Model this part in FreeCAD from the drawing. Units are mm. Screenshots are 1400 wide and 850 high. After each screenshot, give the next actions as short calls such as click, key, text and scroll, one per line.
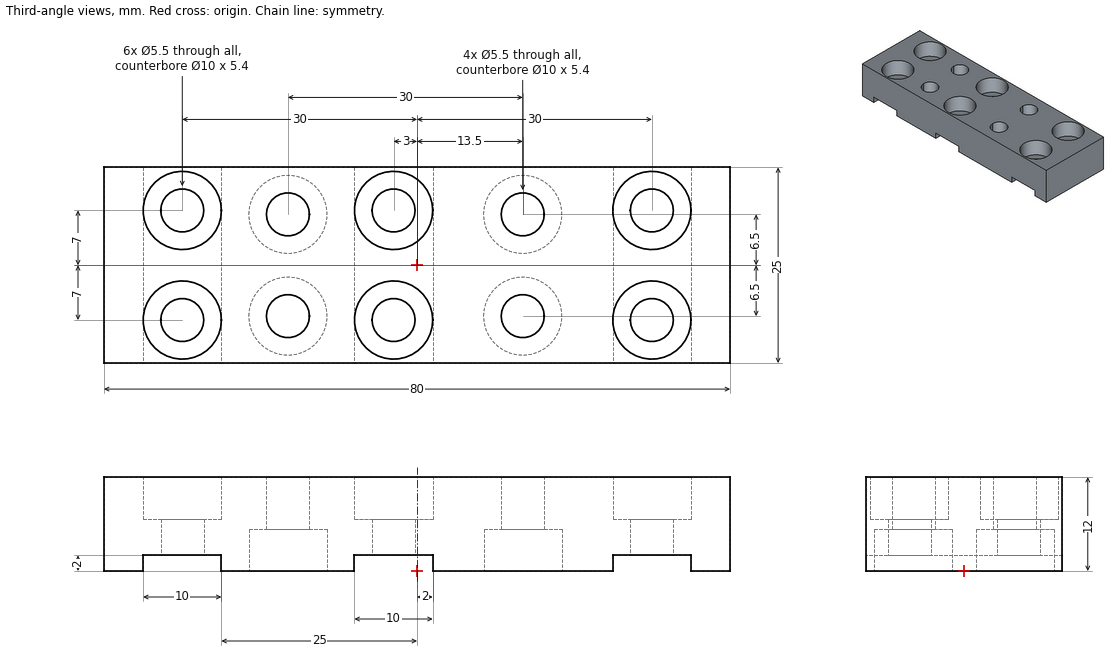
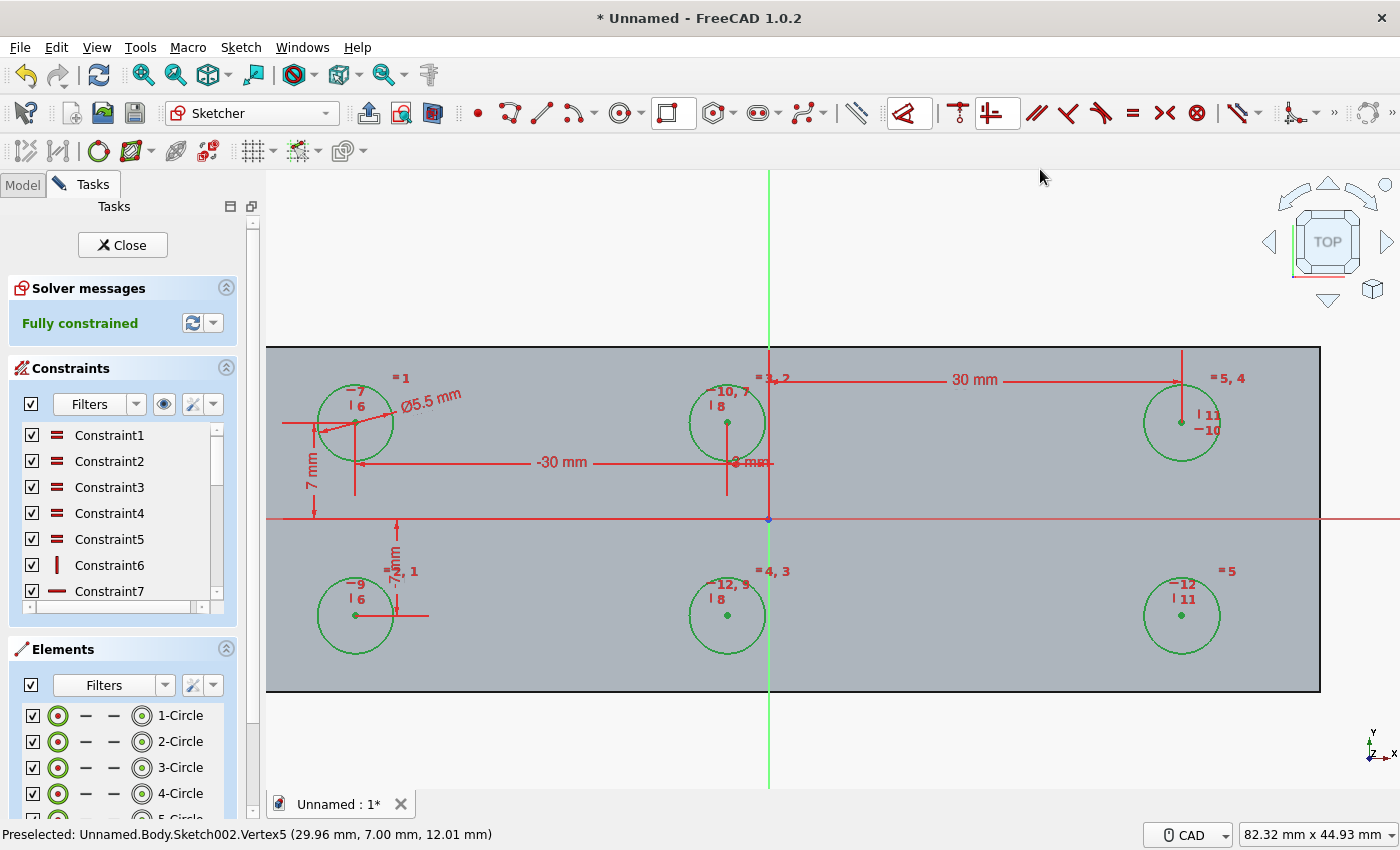
click(123, 245)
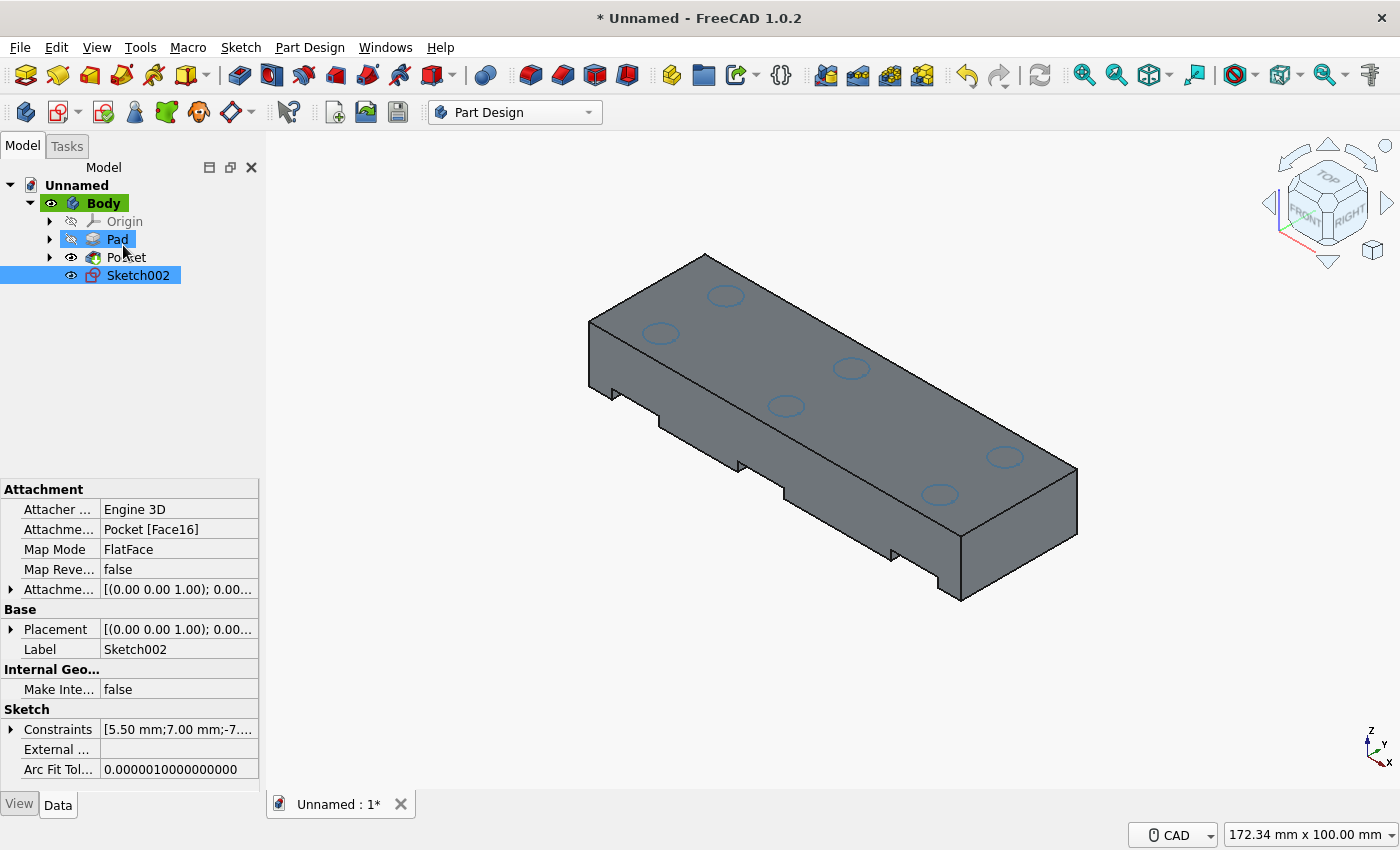
click(272, 76)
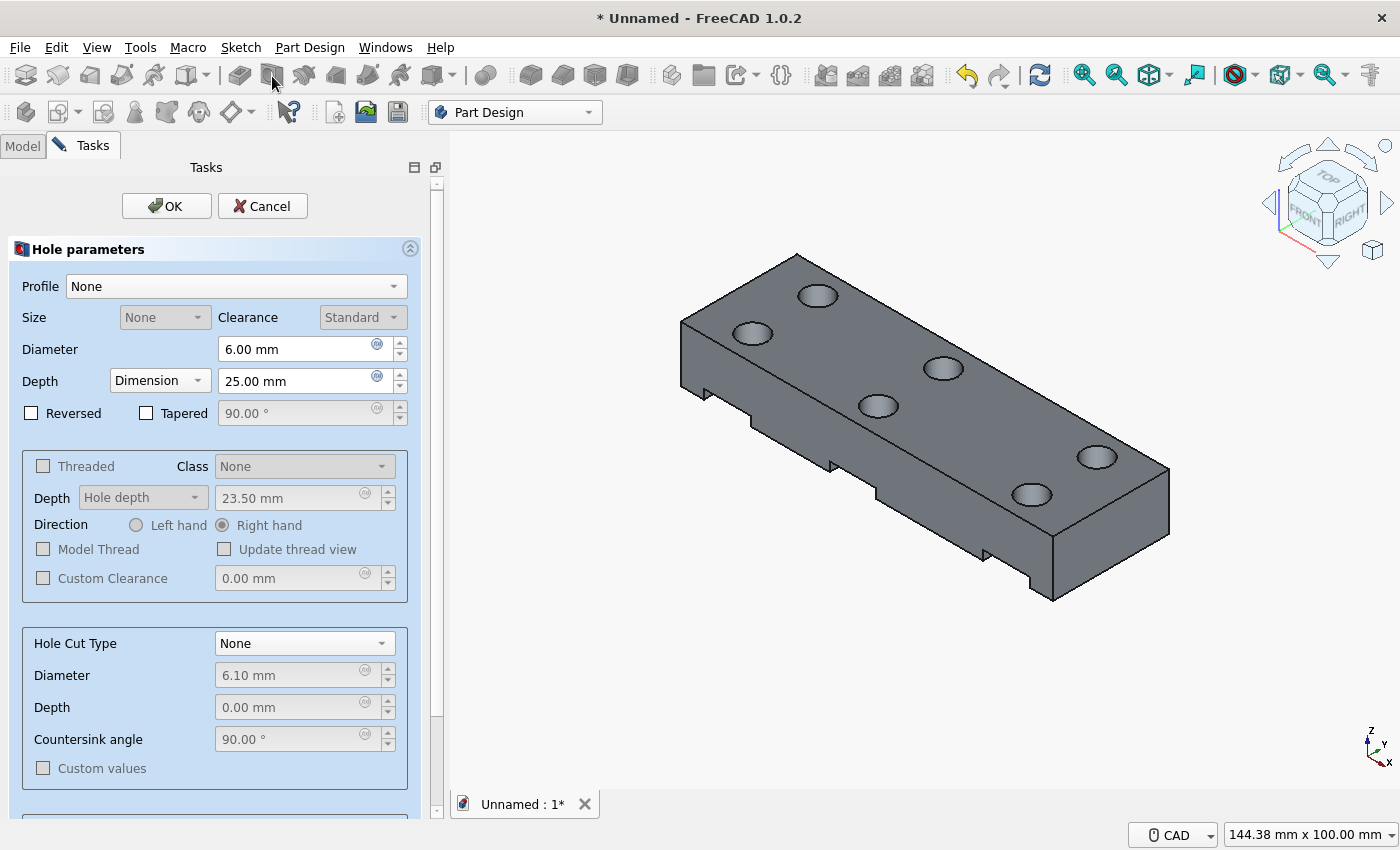
triple_click(305, 349)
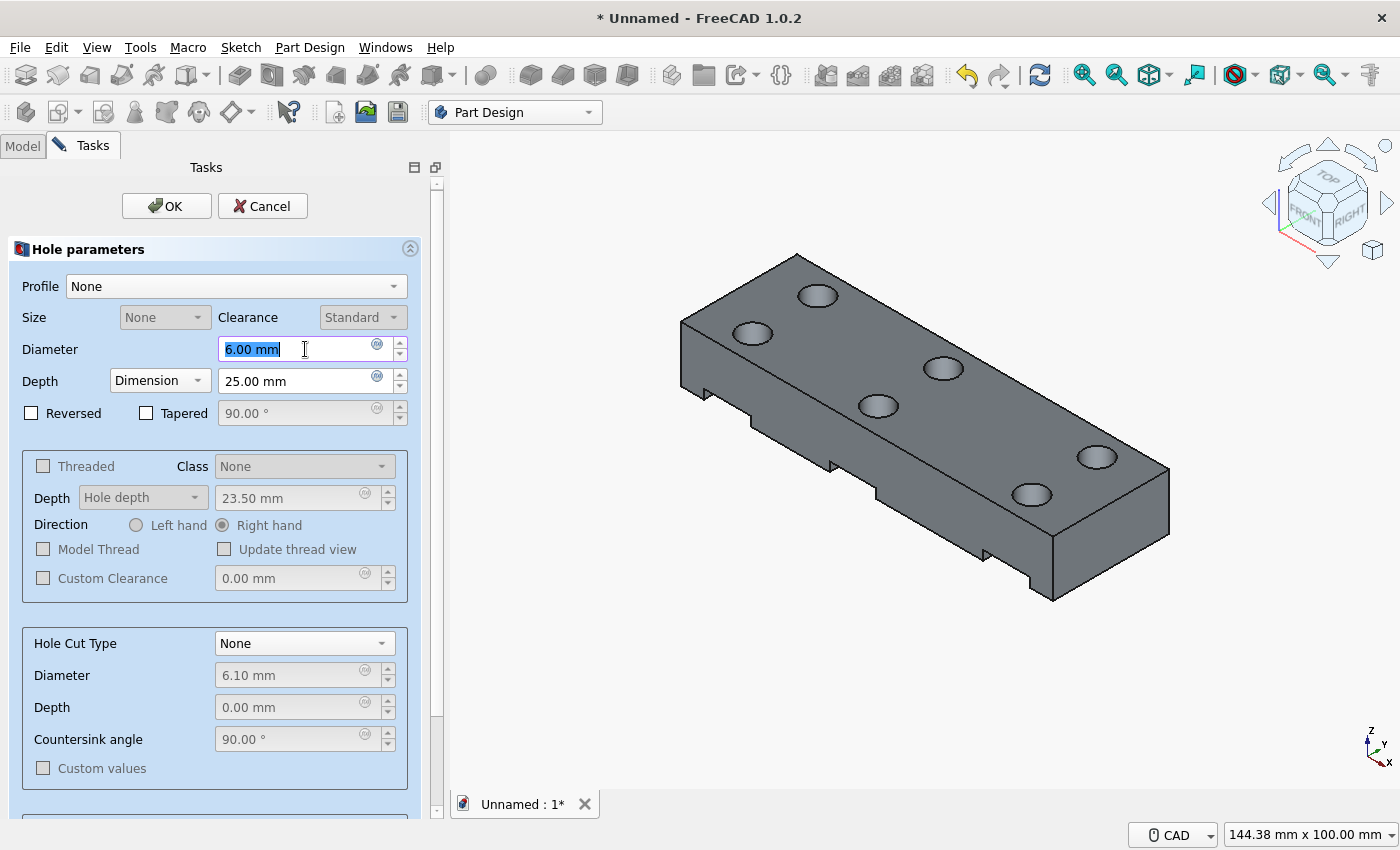
text(5.5)
key(Tab)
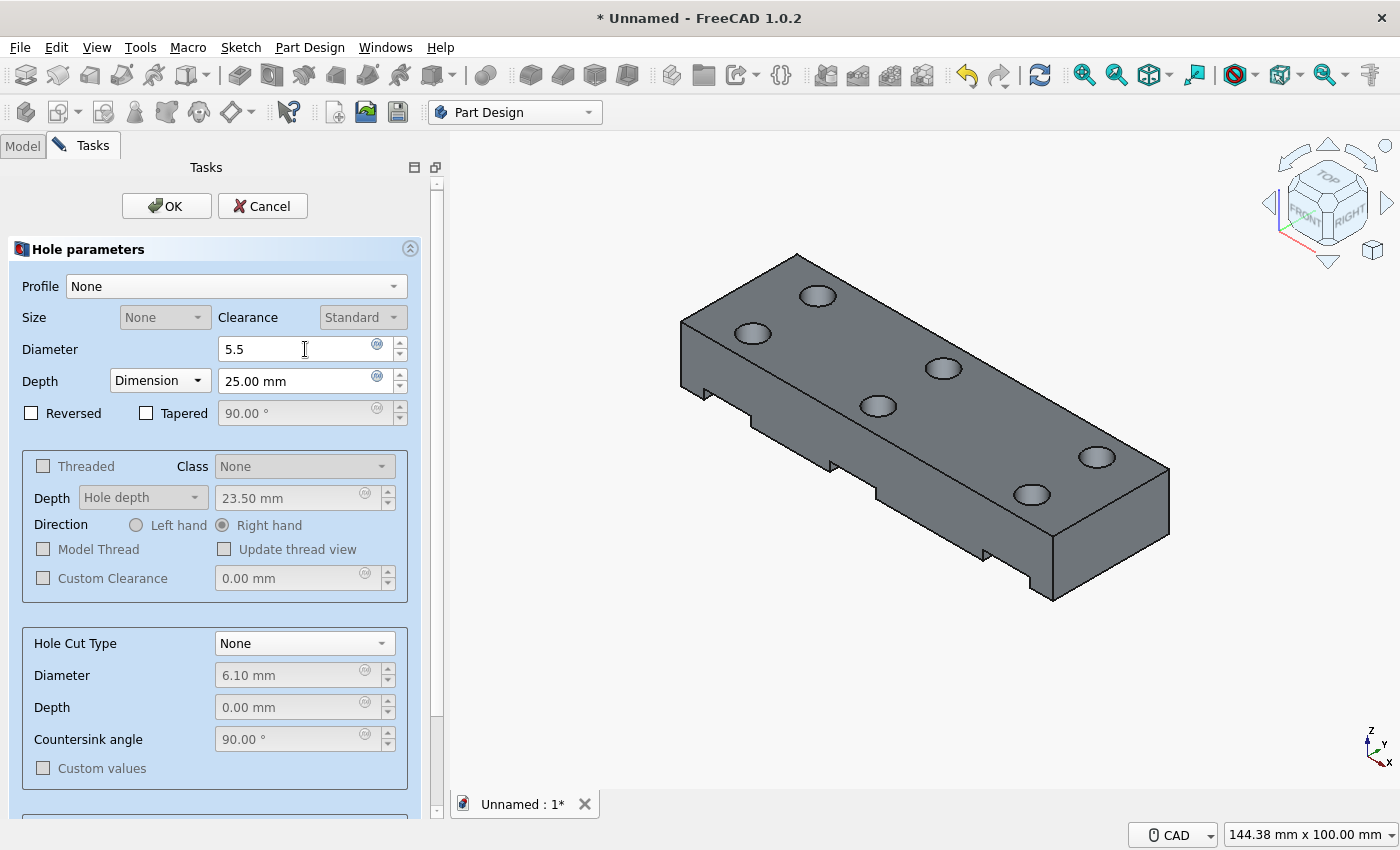
click(161, 380)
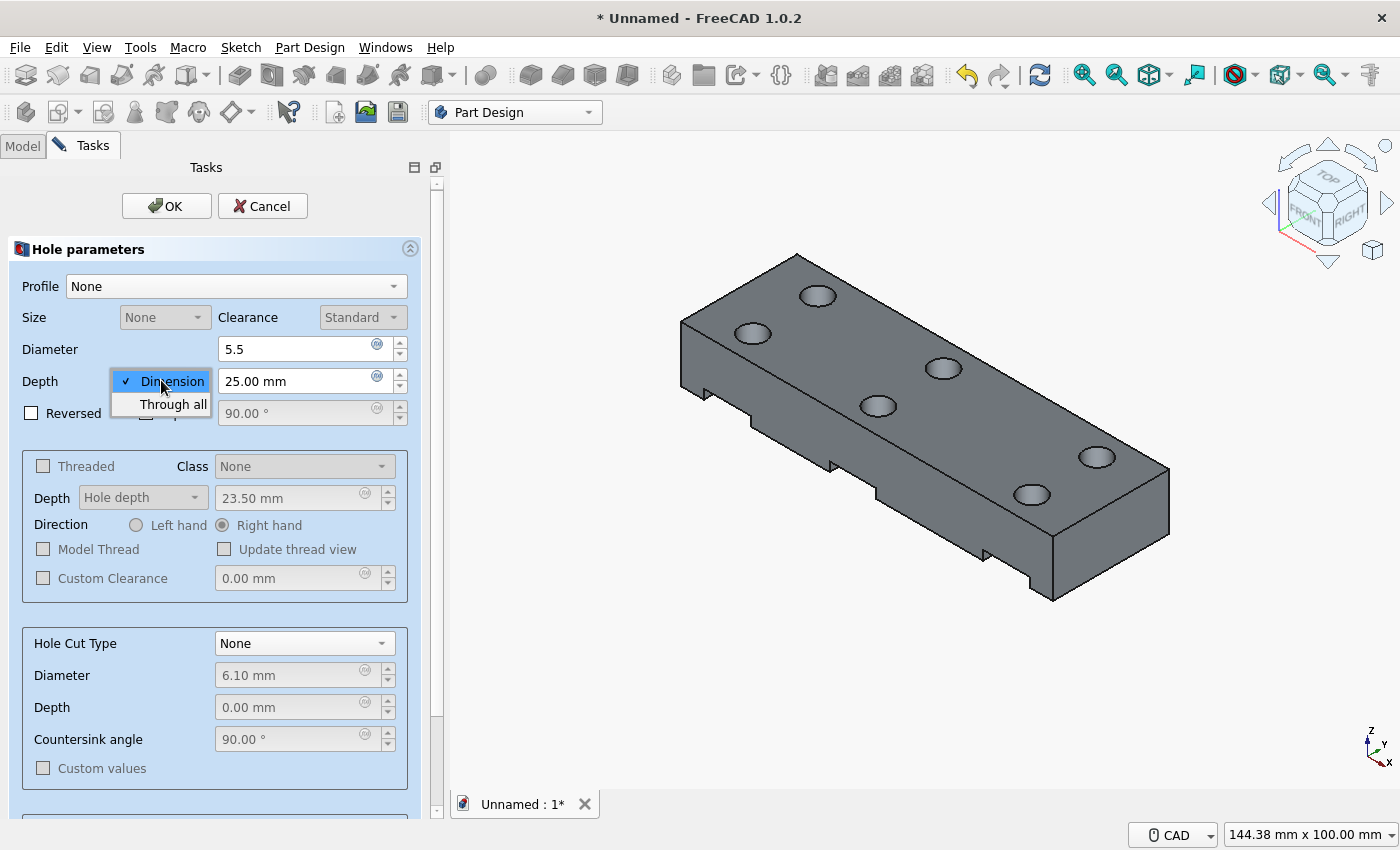
click(160, 404)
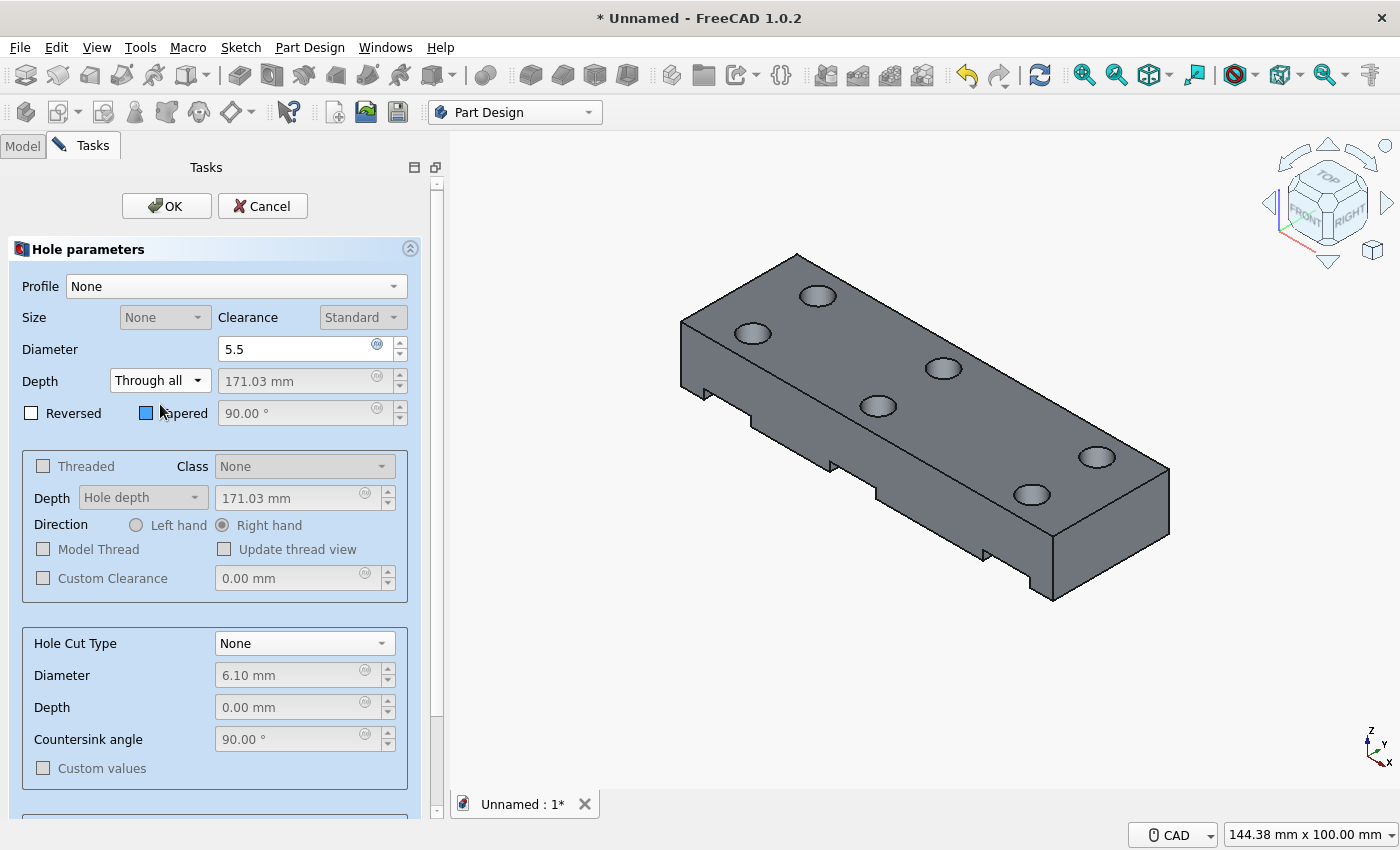
click(306, 644)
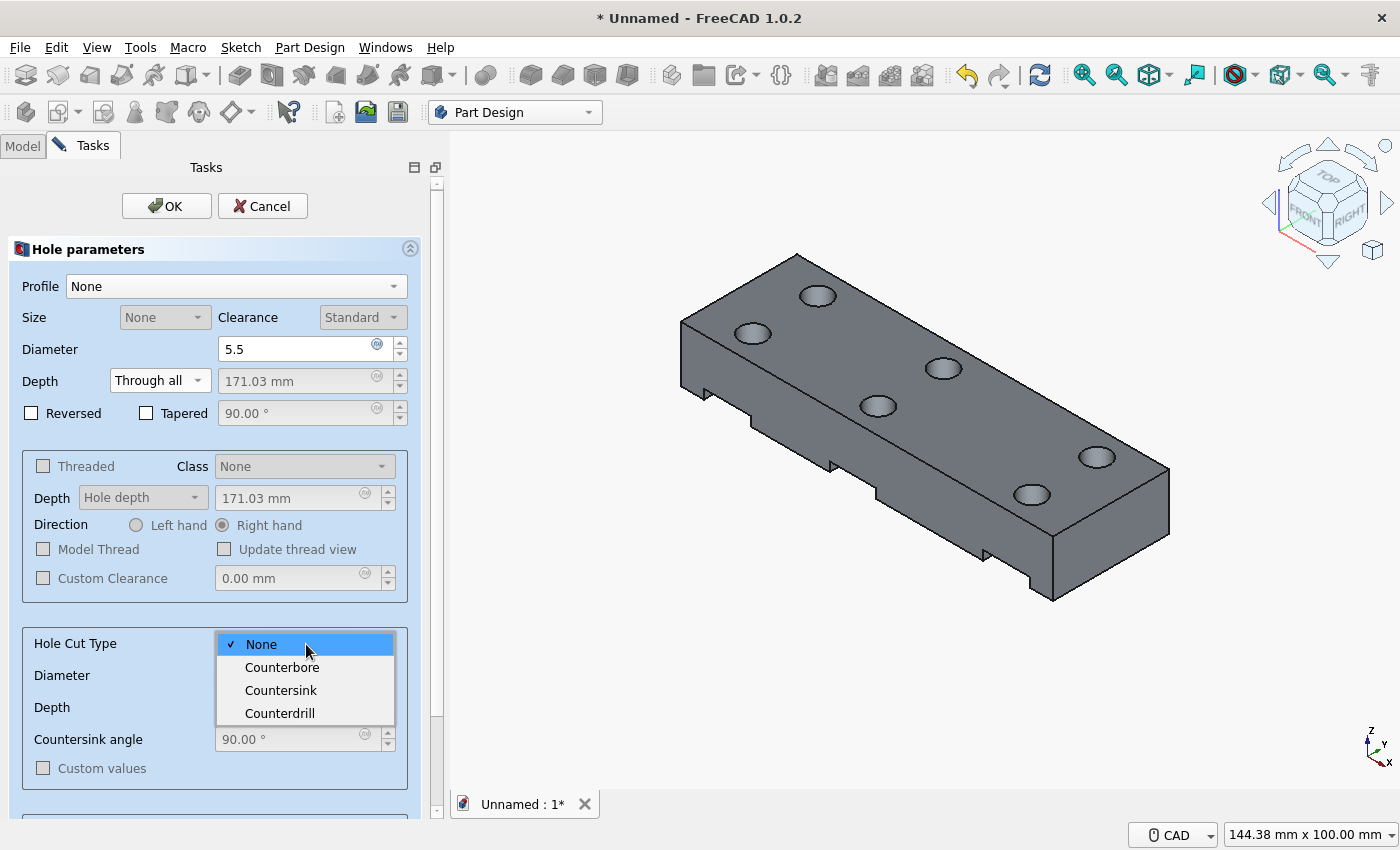
click(304, 668)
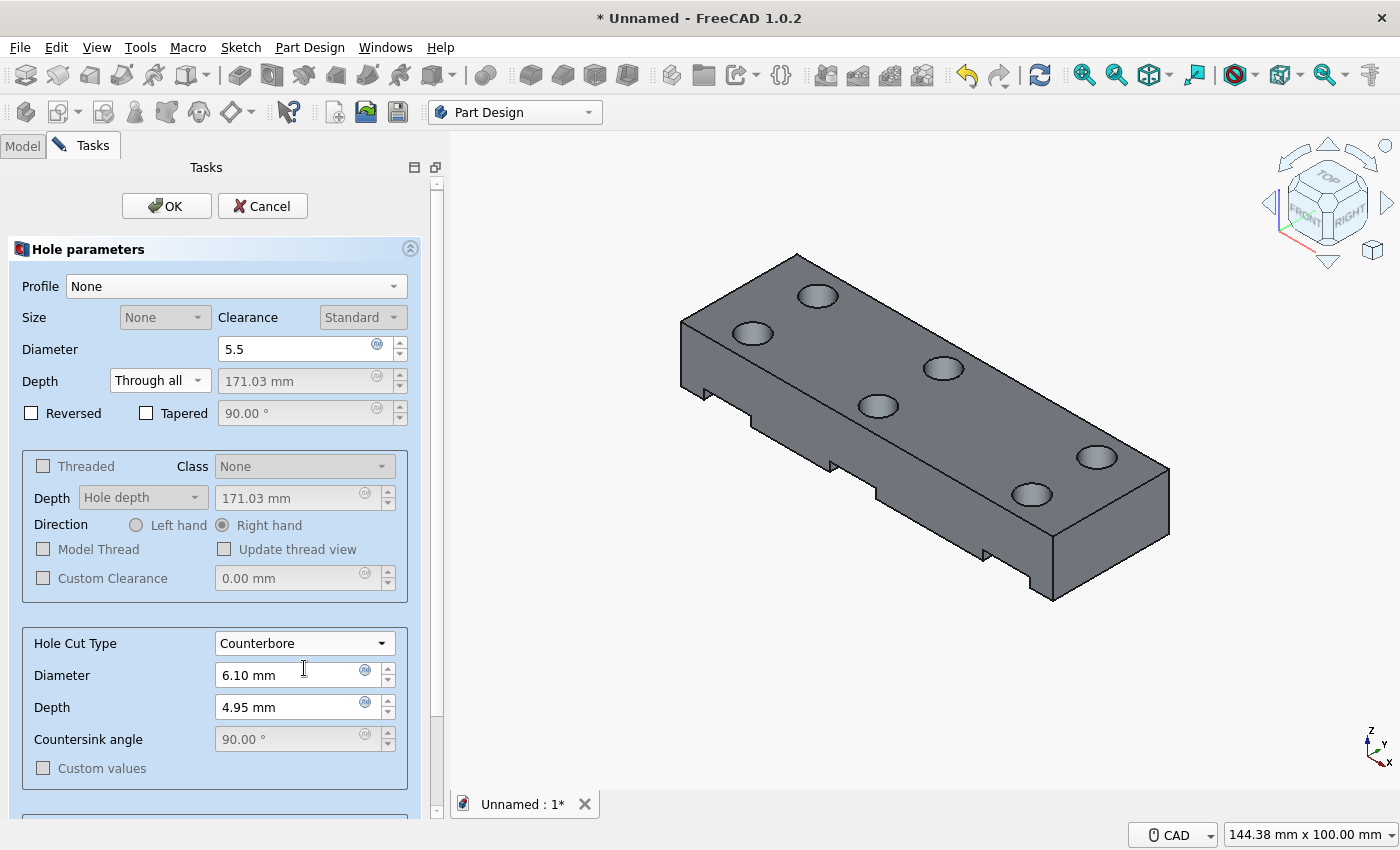
triple_click(298, 675)